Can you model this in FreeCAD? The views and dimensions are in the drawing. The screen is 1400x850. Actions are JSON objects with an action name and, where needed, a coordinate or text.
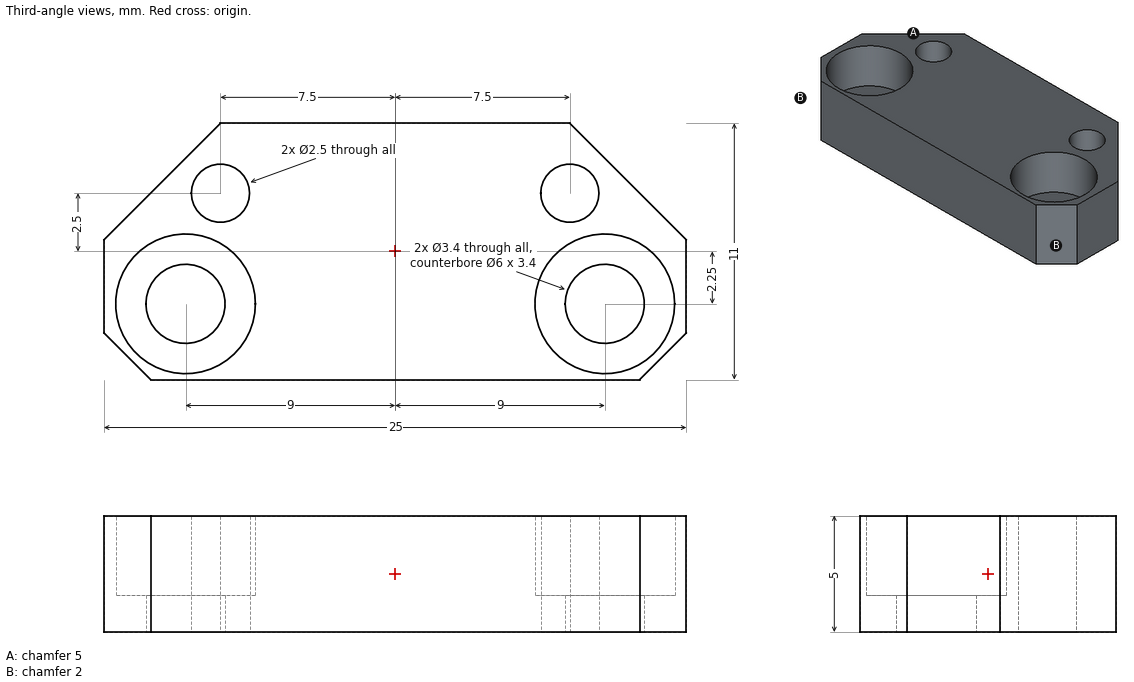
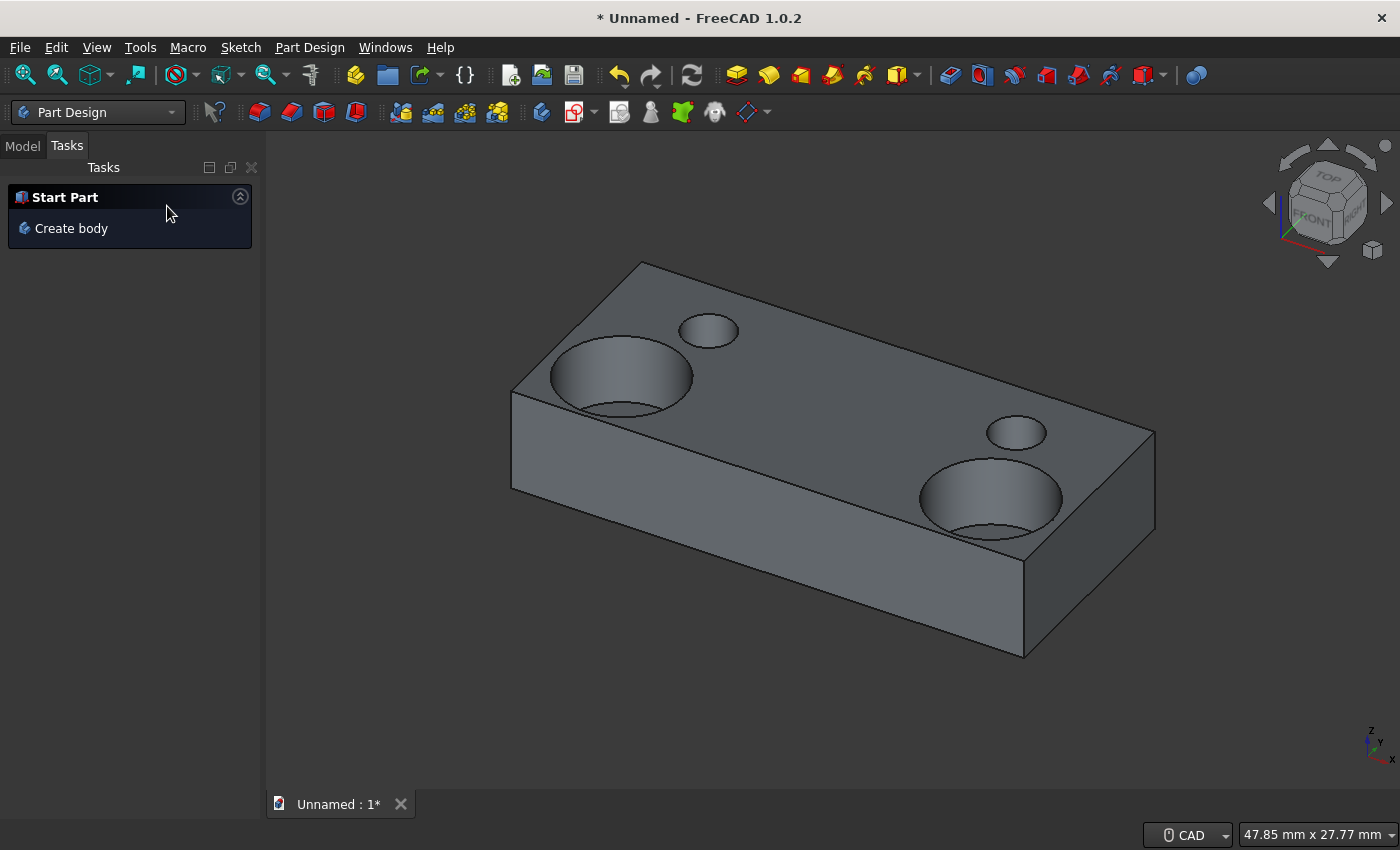
{"action": "key", "text": "0"}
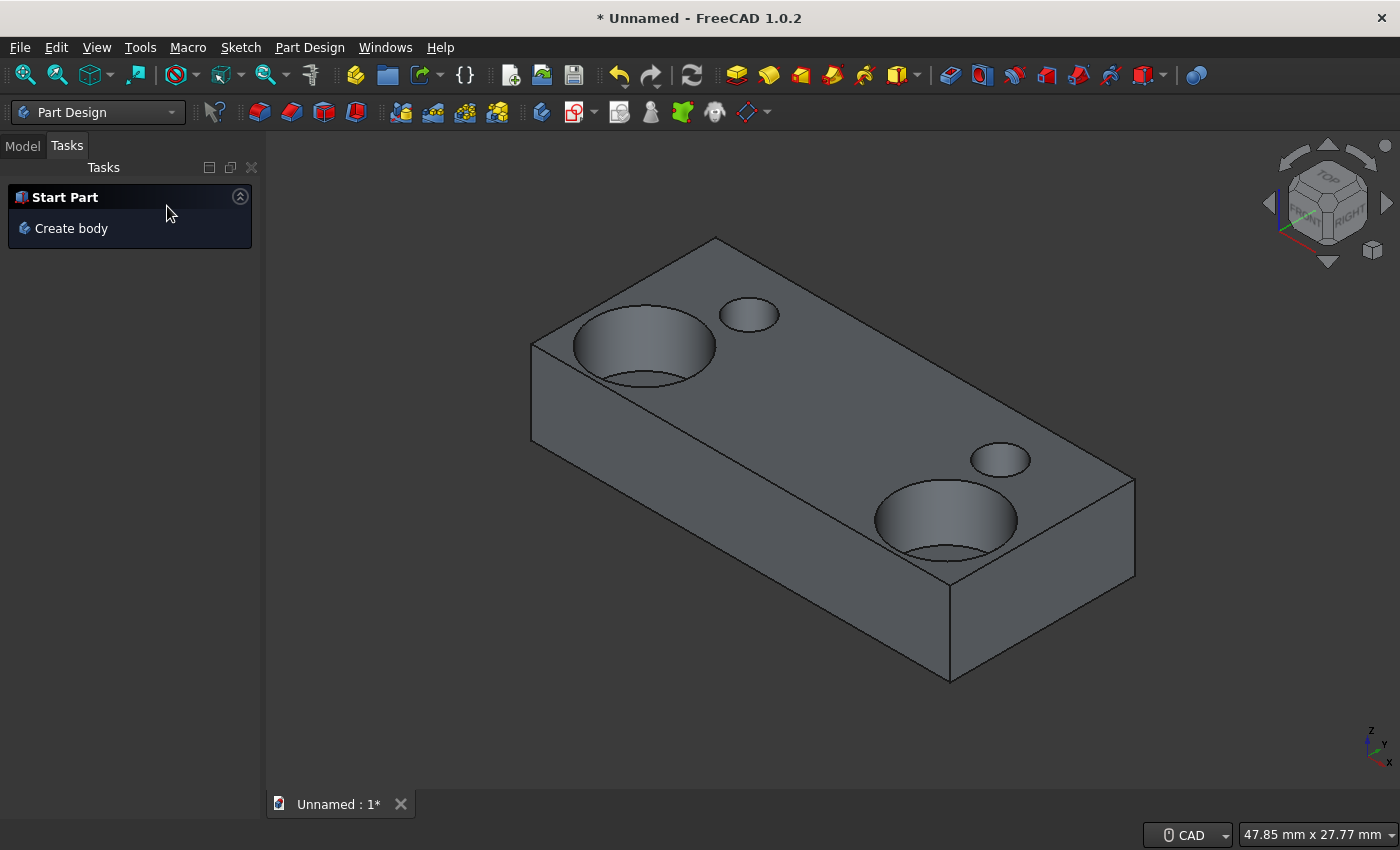
{"action": "key", "text": "2"}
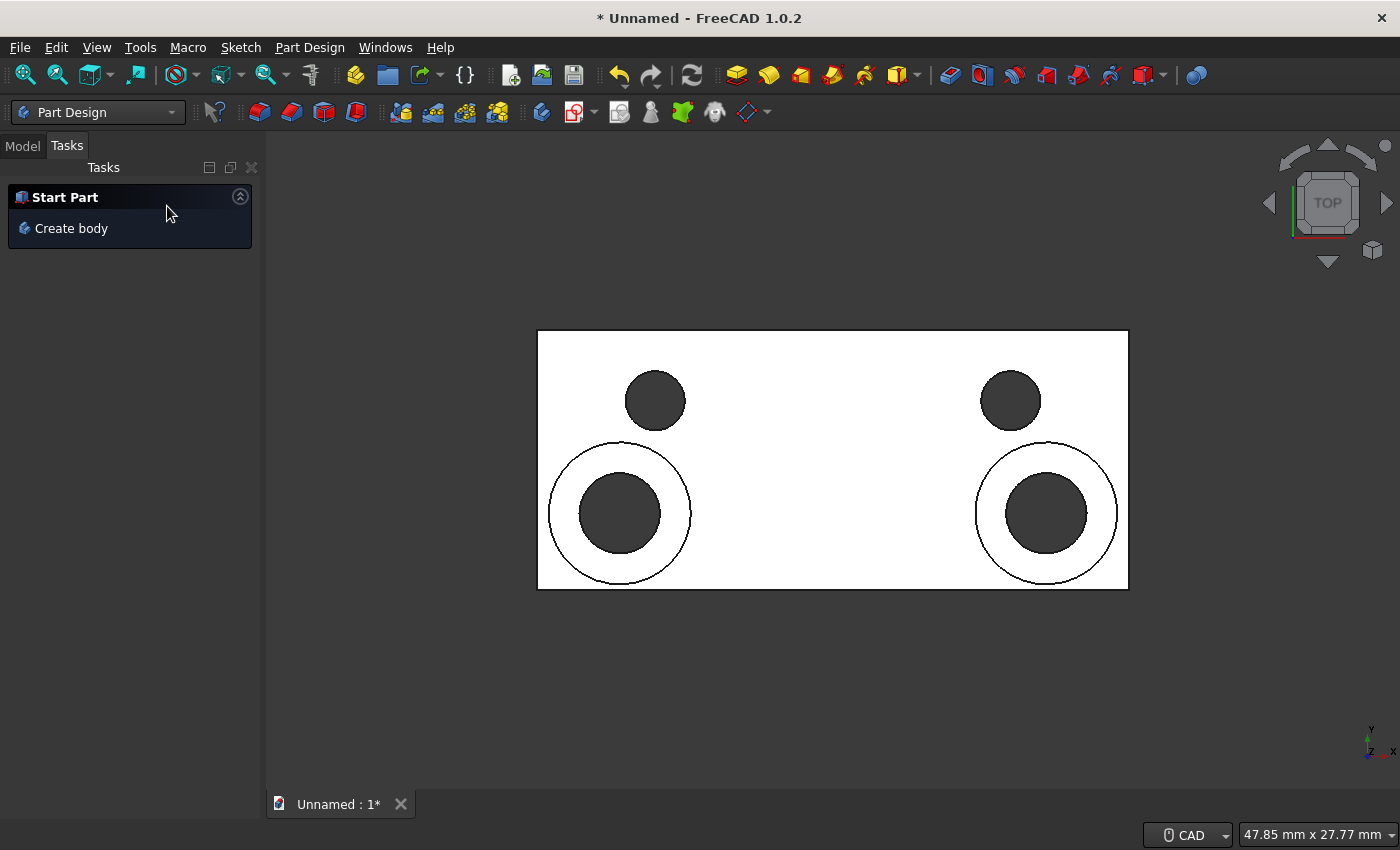
{"action": "key", "text": "1"}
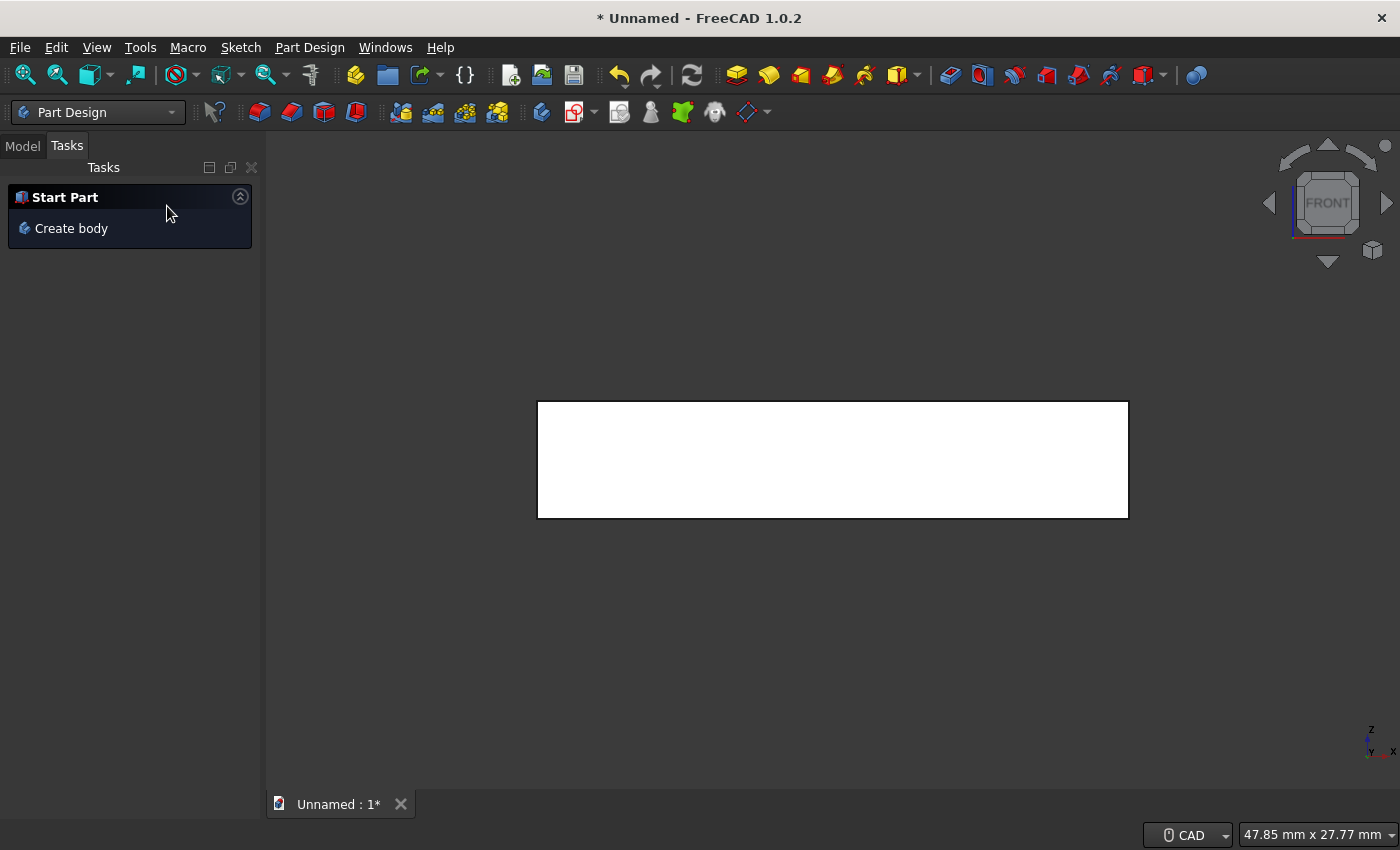
{"action": "key", "text": "3"}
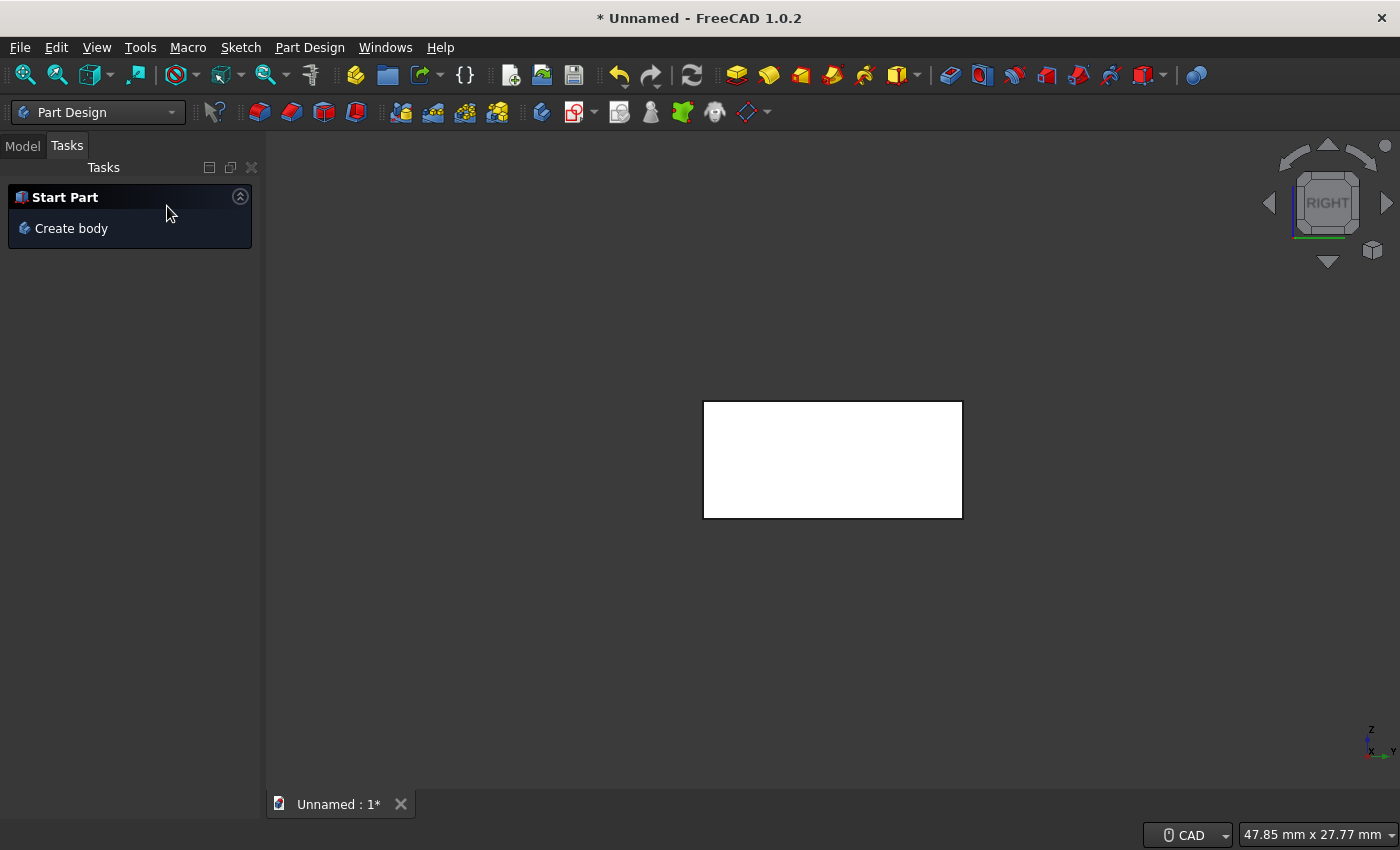
{"action": "key", "text": "v f"}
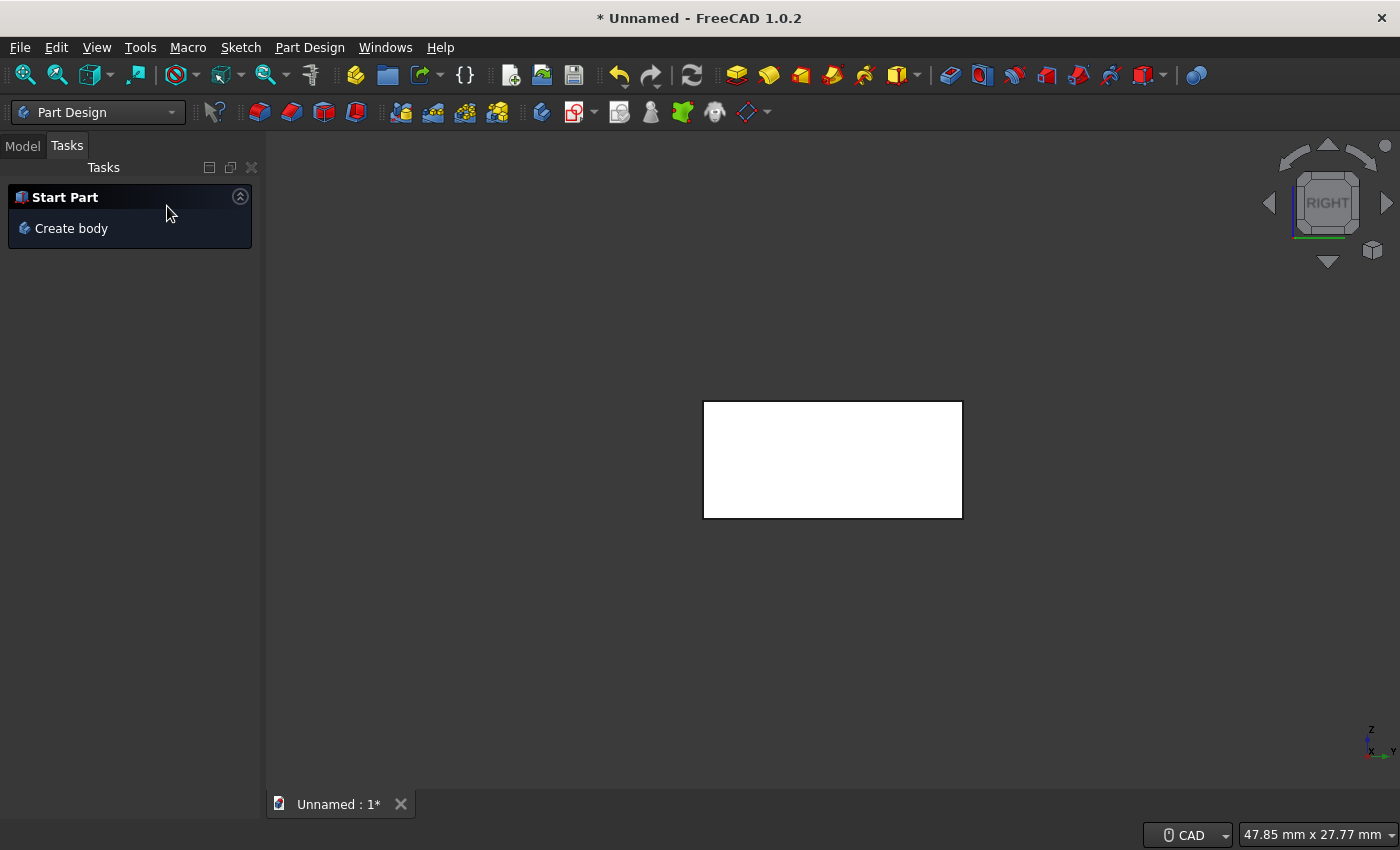
{"action": "left_click", "coordinate": [963, 459]}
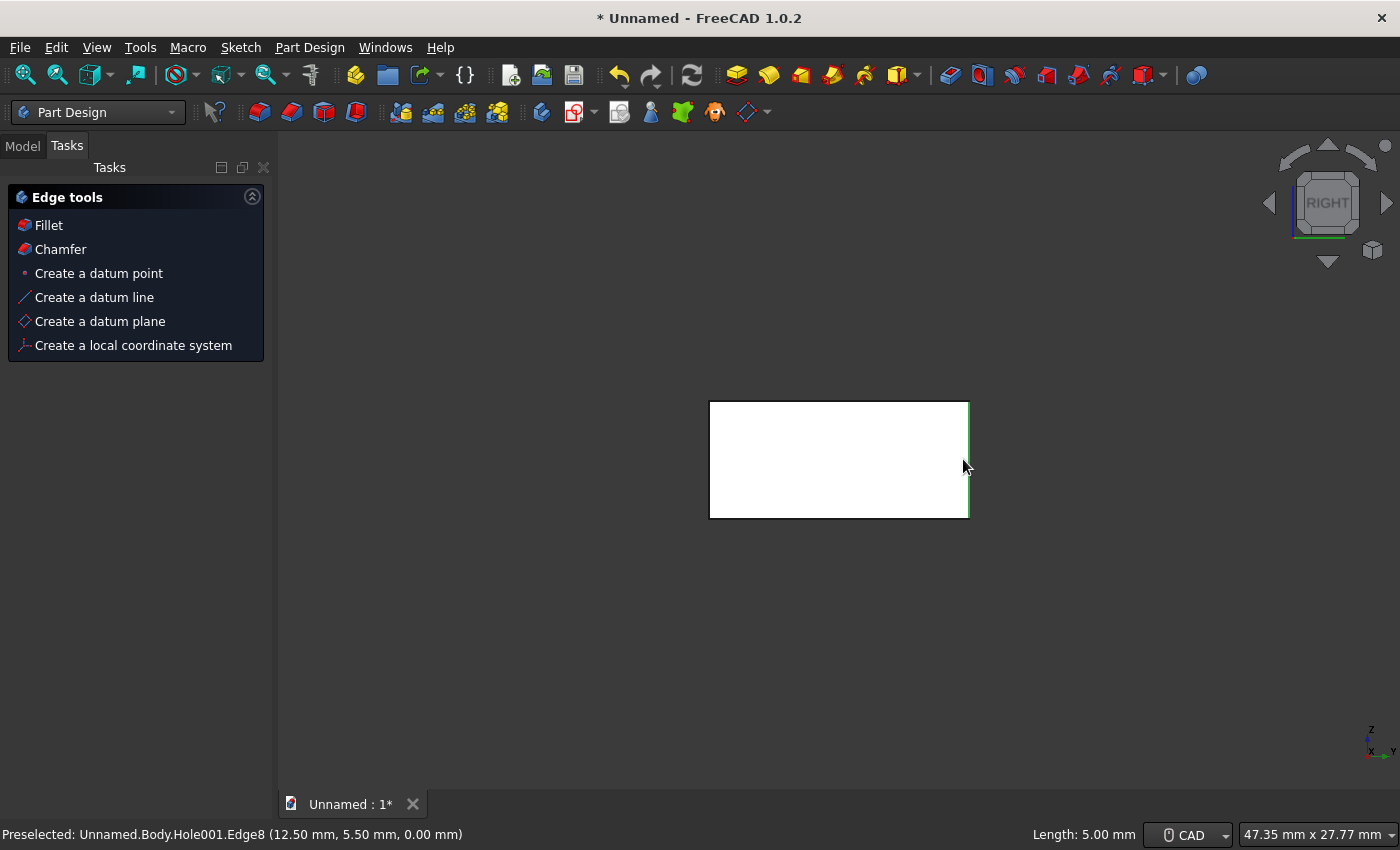
{"action": "key", "text": "5"}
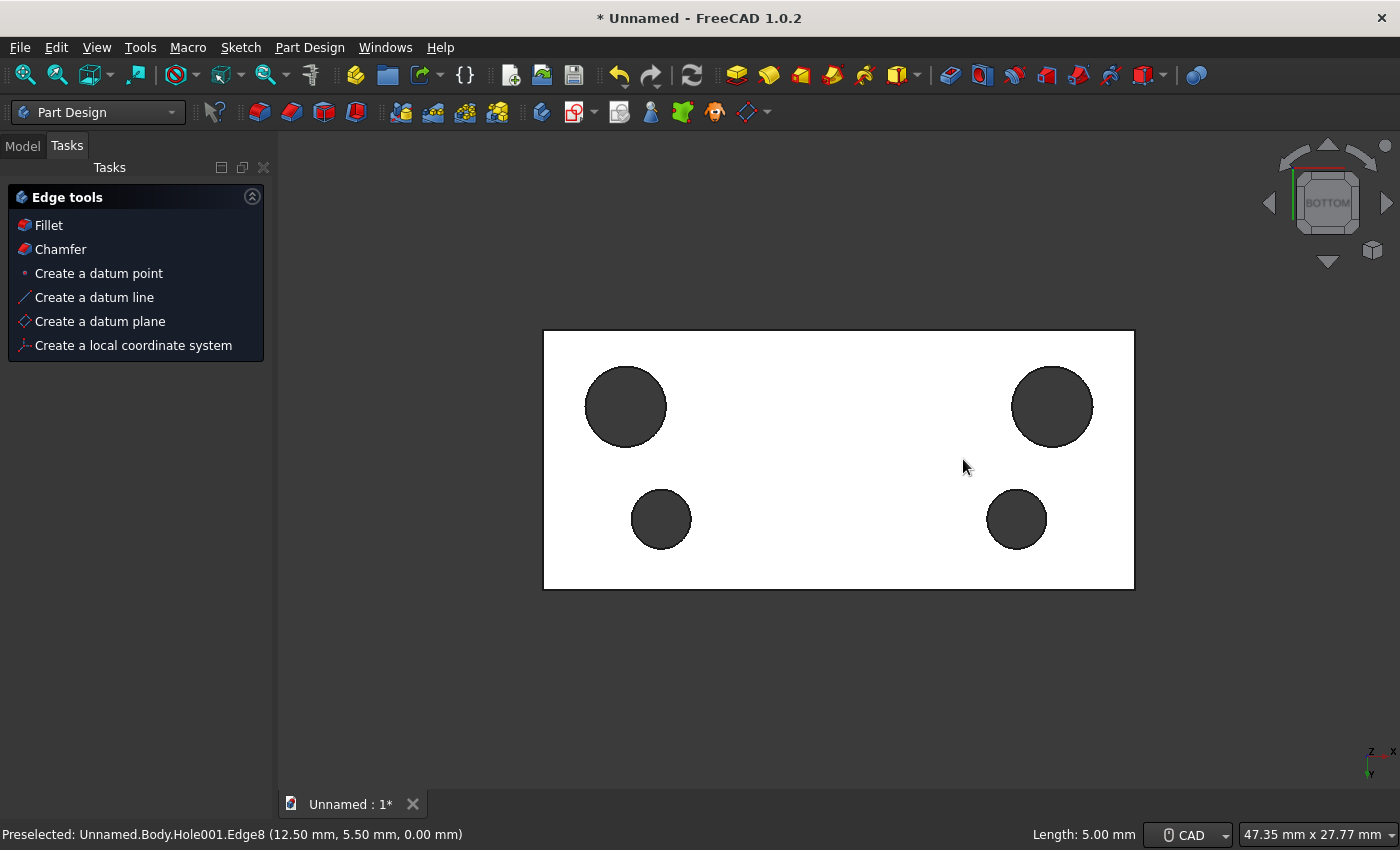
{"action": "key", "text": "4"}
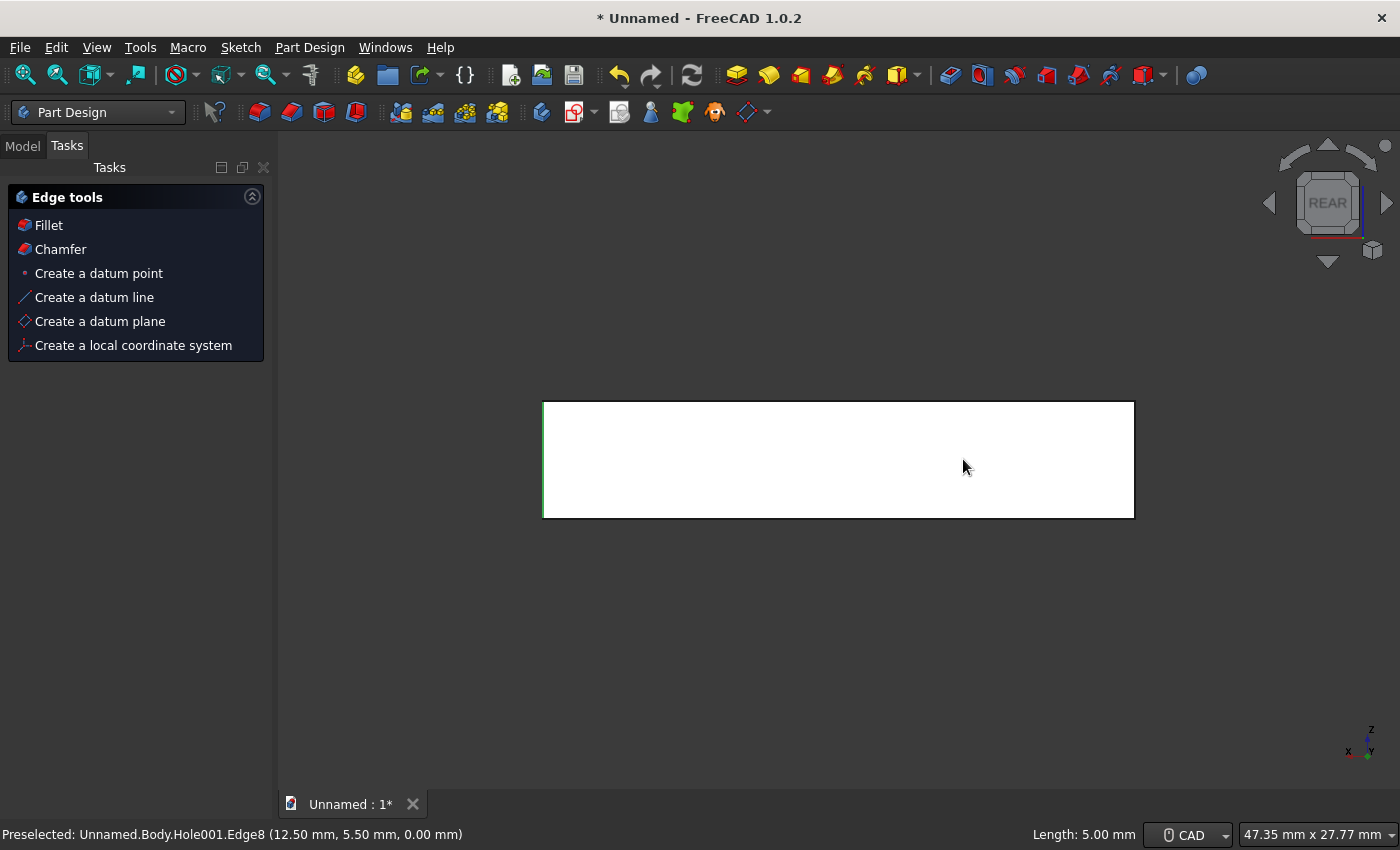
{"action": "left_click", "coordinate": [1135, 459], "text": "ctrl"}